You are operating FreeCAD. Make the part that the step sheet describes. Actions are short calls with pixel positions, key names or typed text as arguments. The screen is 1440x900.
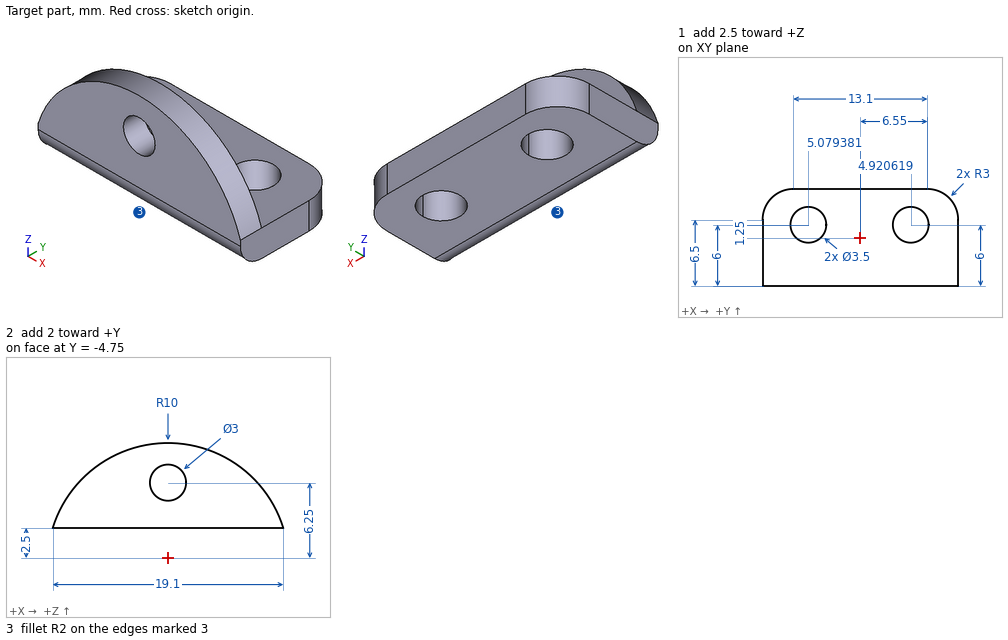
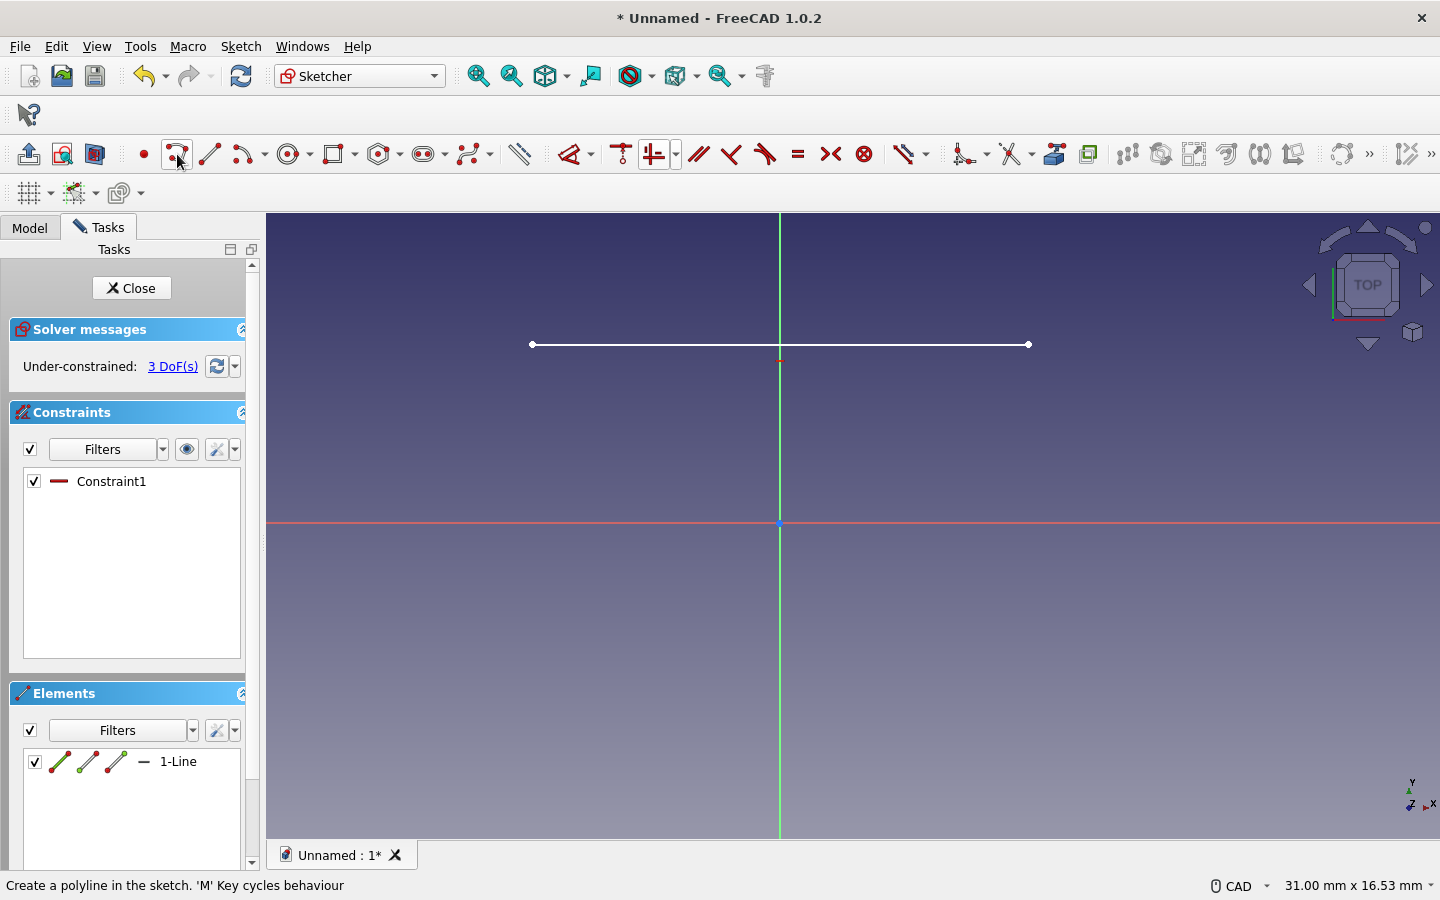
click(418, 457)
click(418, 703)
click(1141, 703)
click(1141, 457)
right_click(1141, 457)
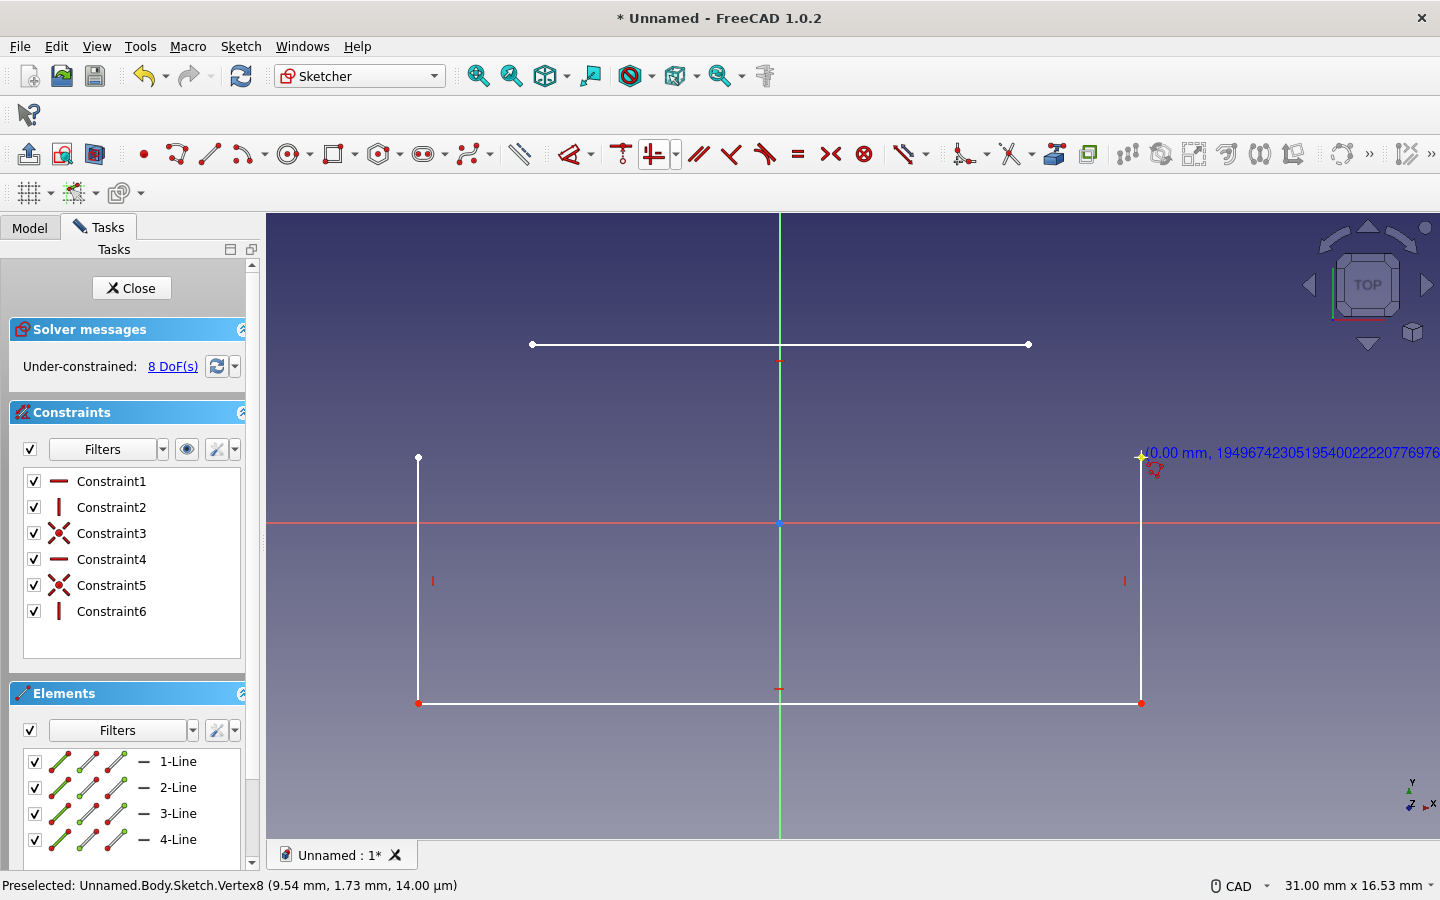
click(264, 154)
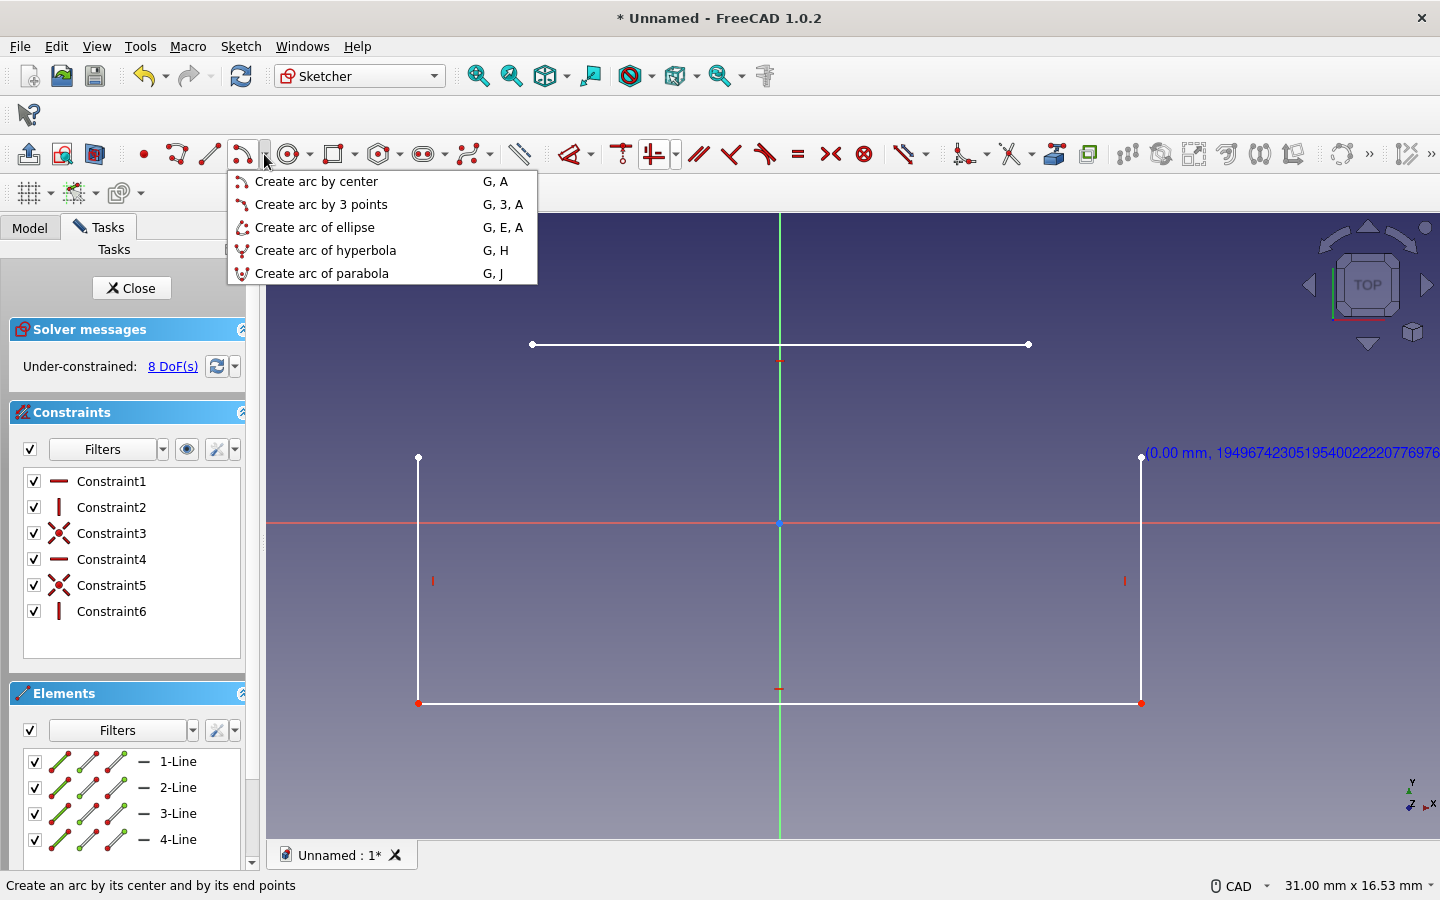
click(382, 204)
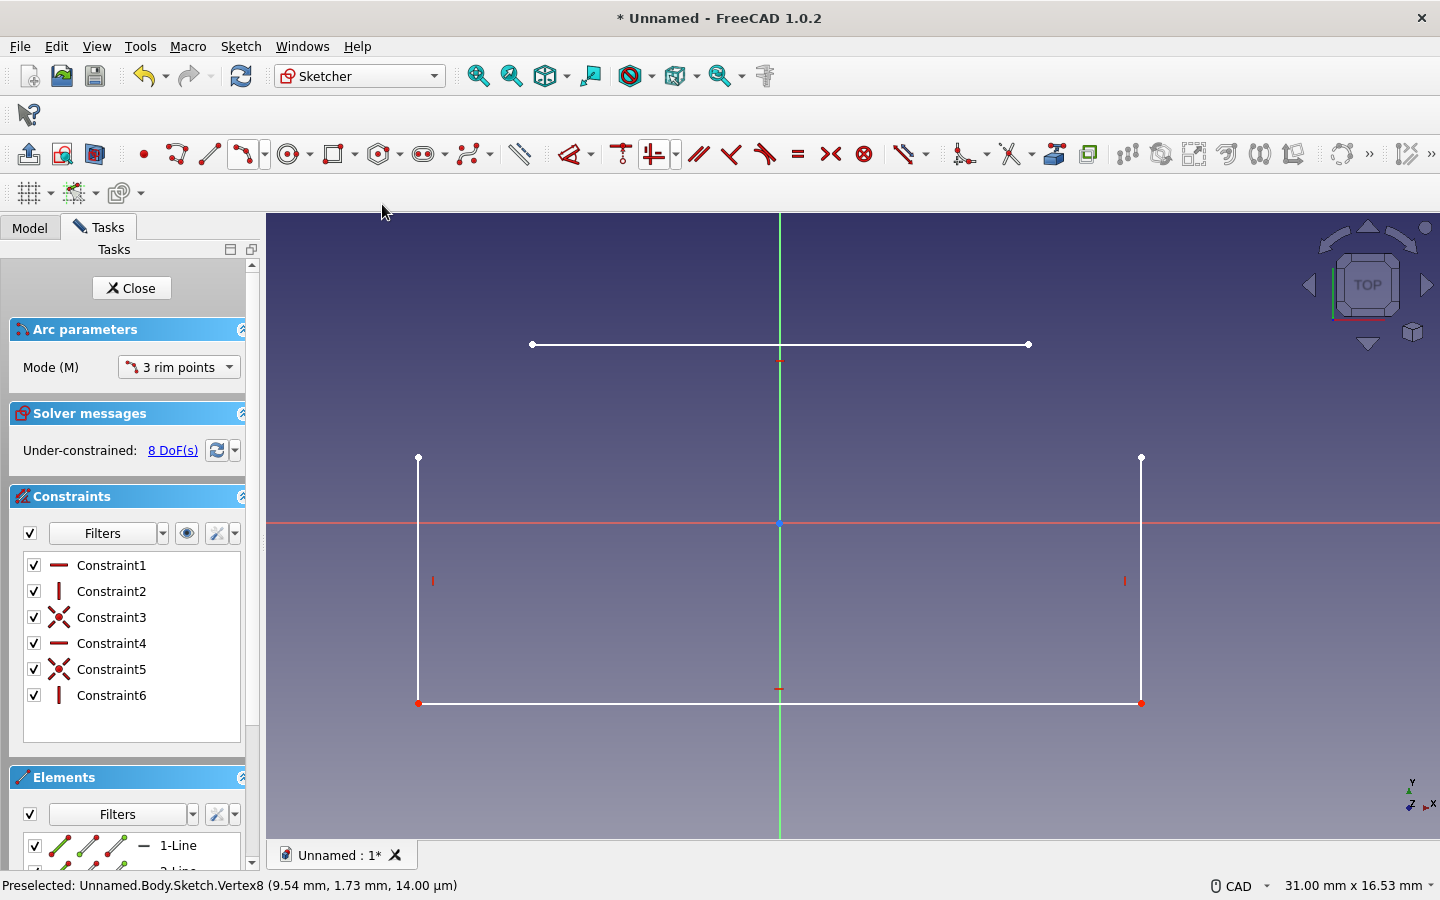
click(532, 345)
click(418, 458)
click(451, 377)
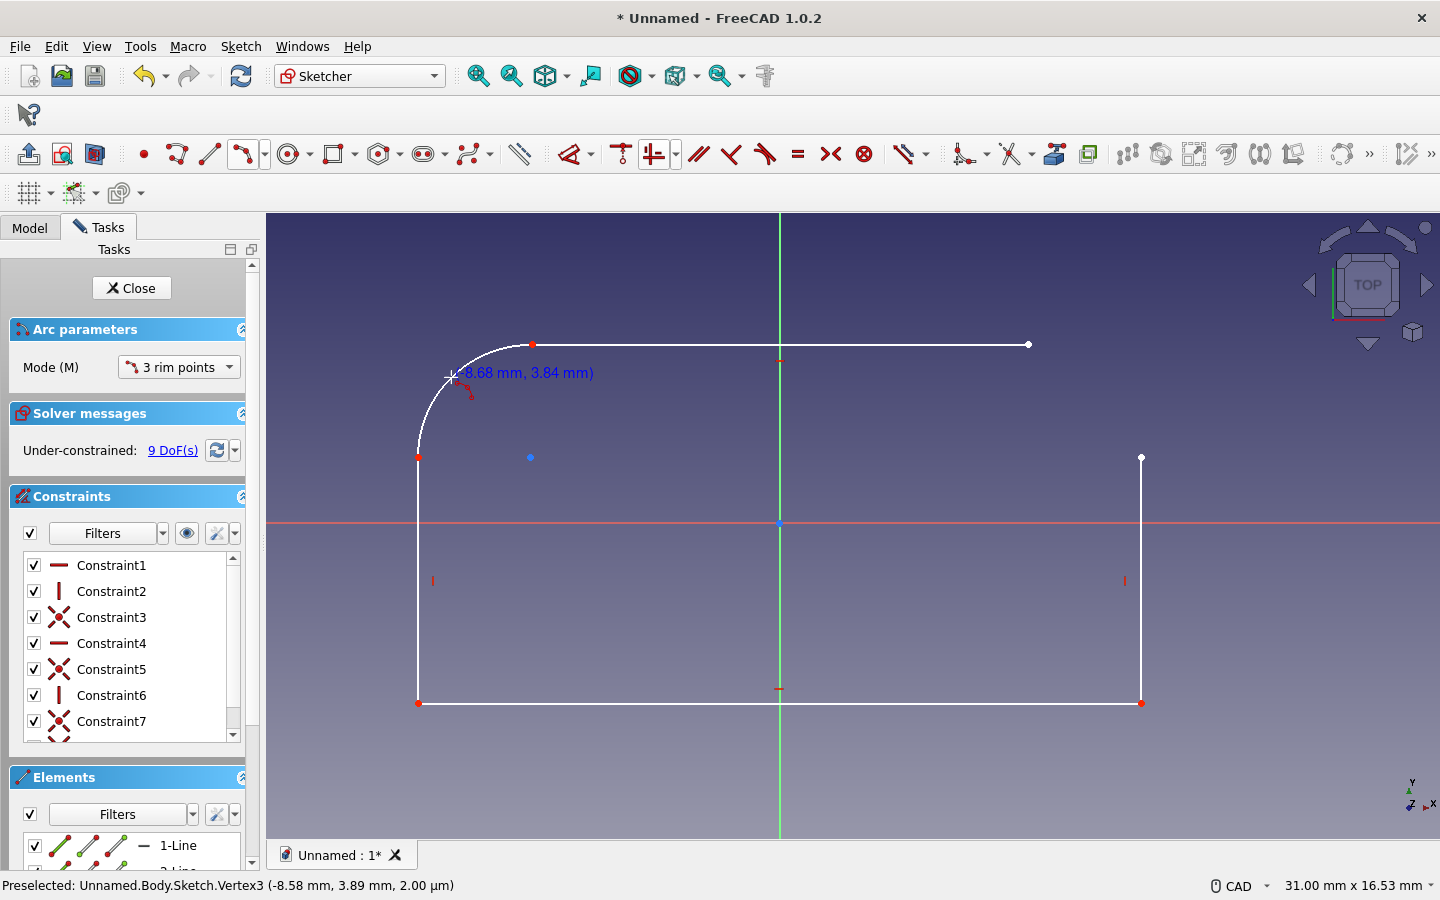
click(1141, 458)
click(1028, 345)
click(1108, 377)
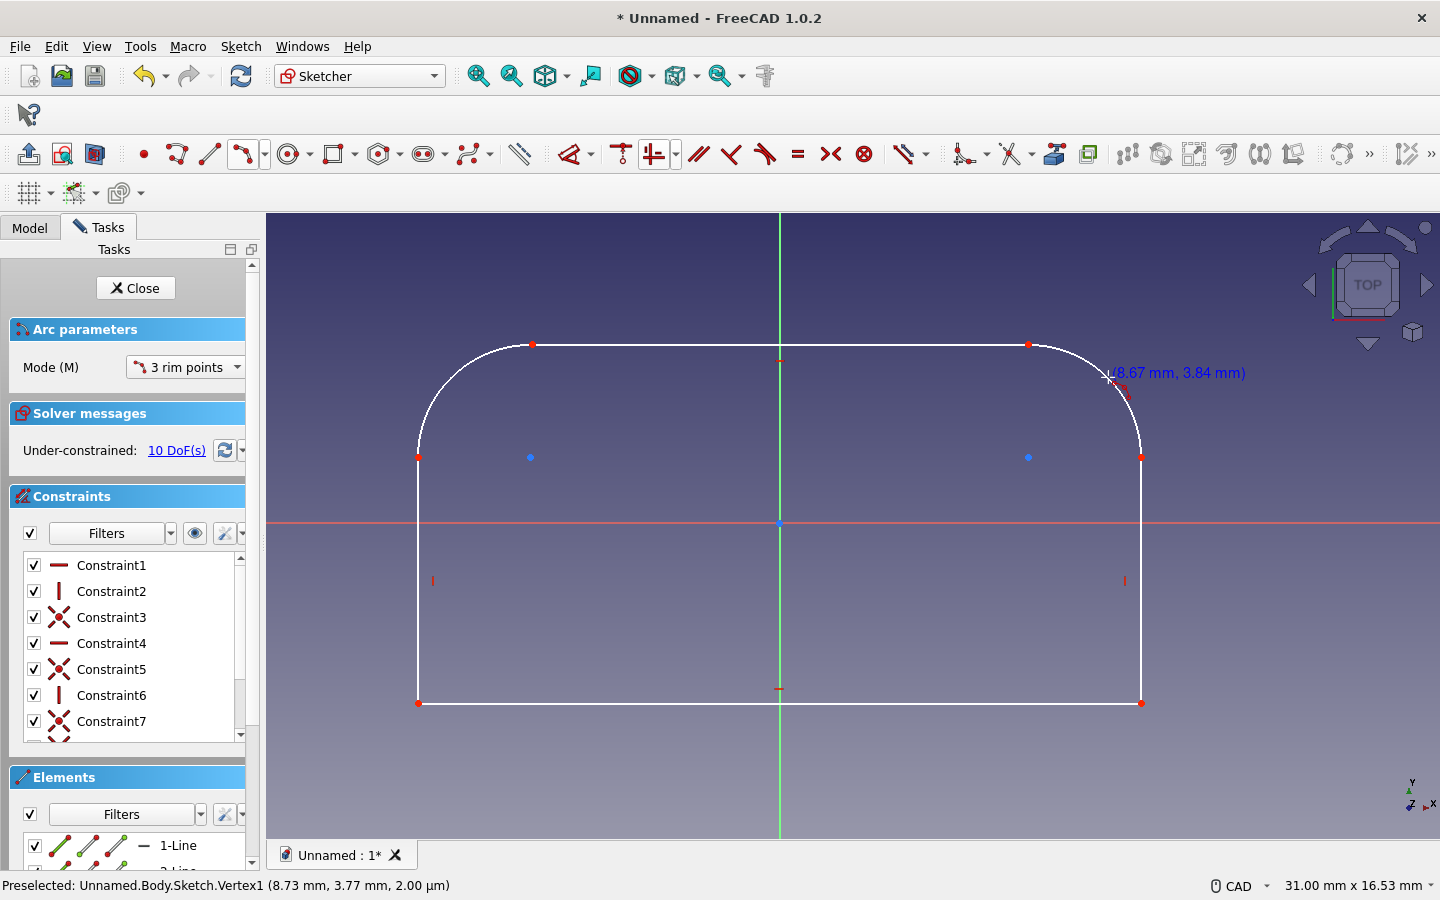
click(288, 154)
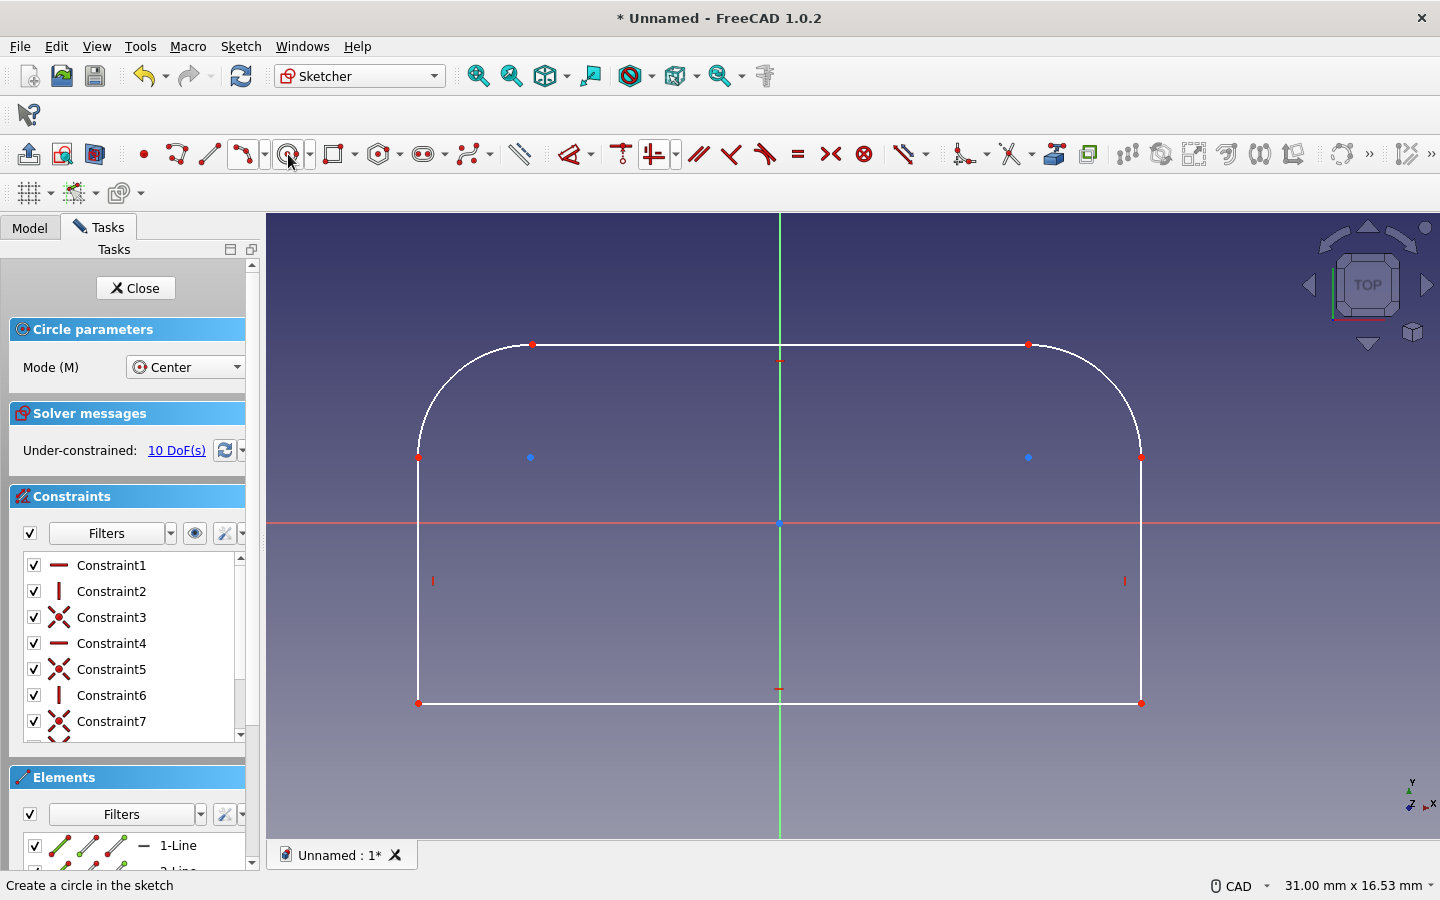
click(587, 476)
click(634, 429)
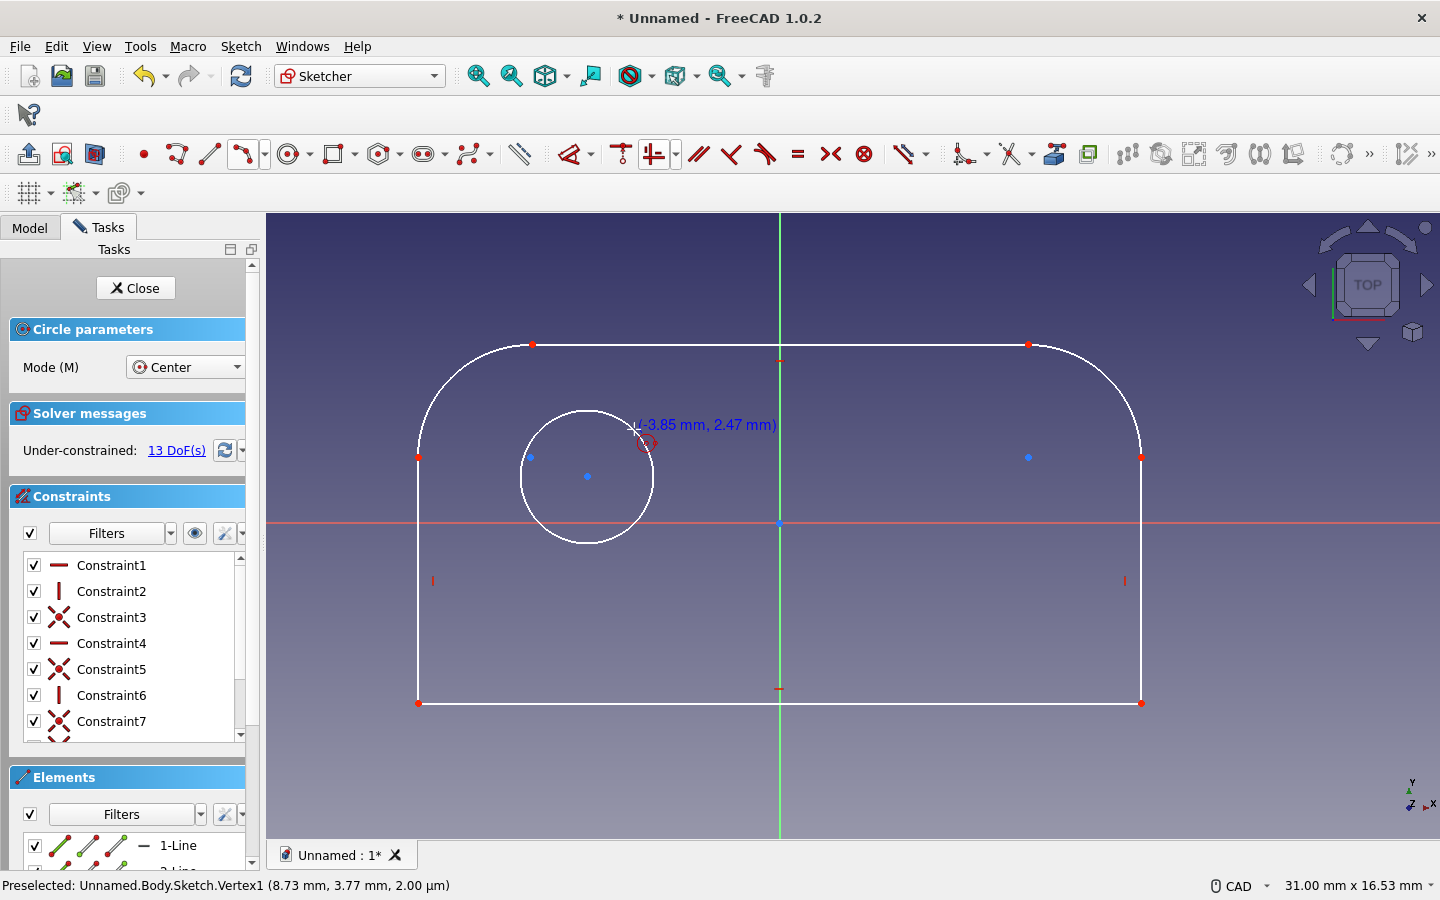
click(966, 476)
click(1013, 429)
key(Escape)